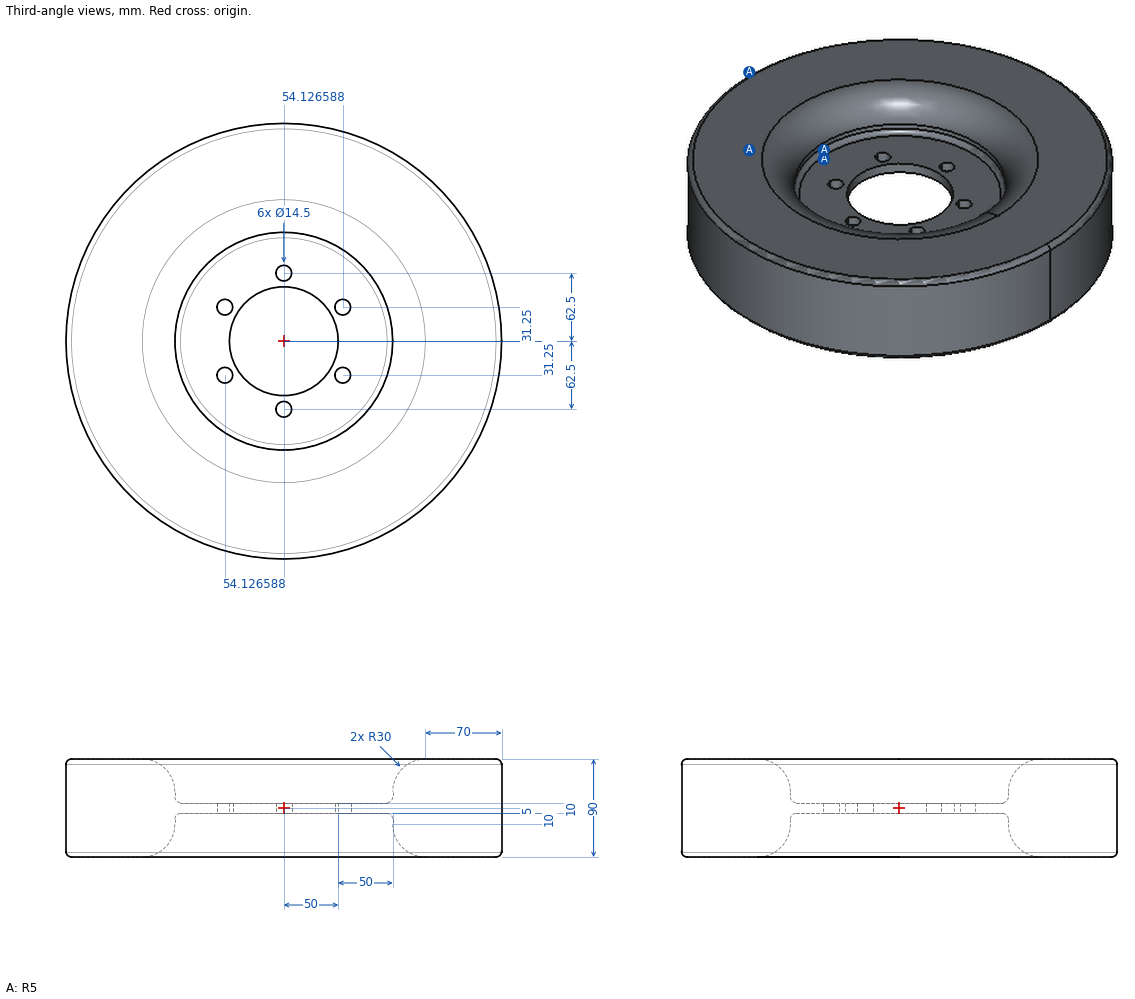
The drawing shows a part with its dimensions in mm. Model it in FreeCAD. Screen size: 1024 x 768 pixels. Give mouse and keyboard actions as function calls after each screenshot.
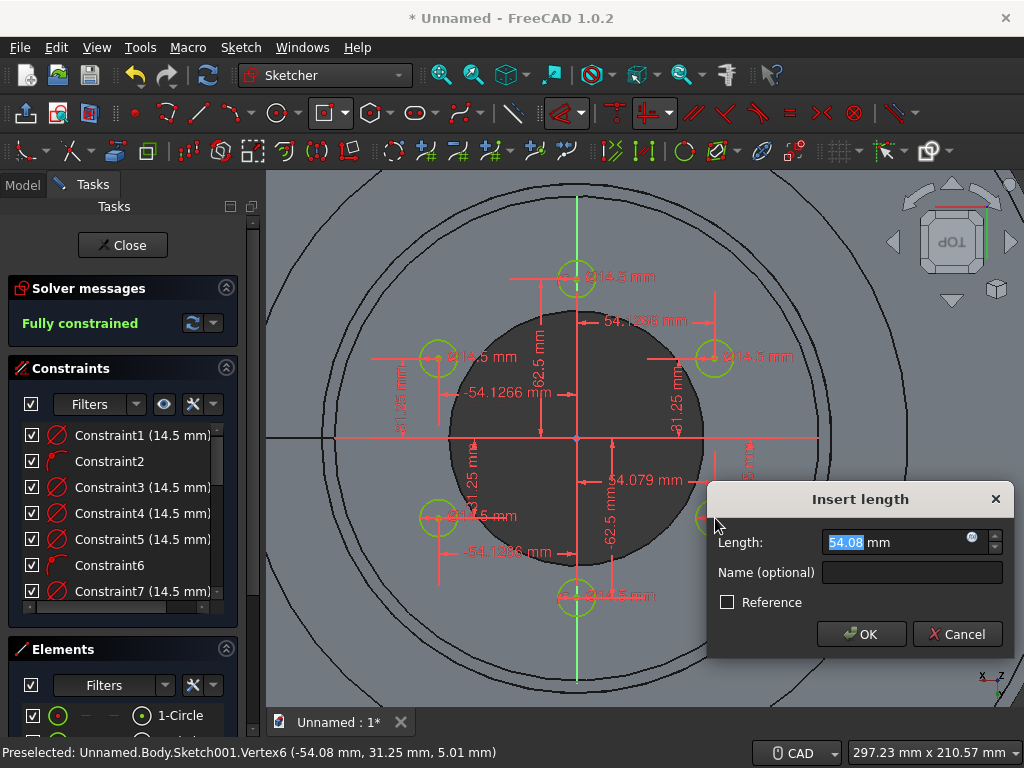
text(54.126588)
key(Return)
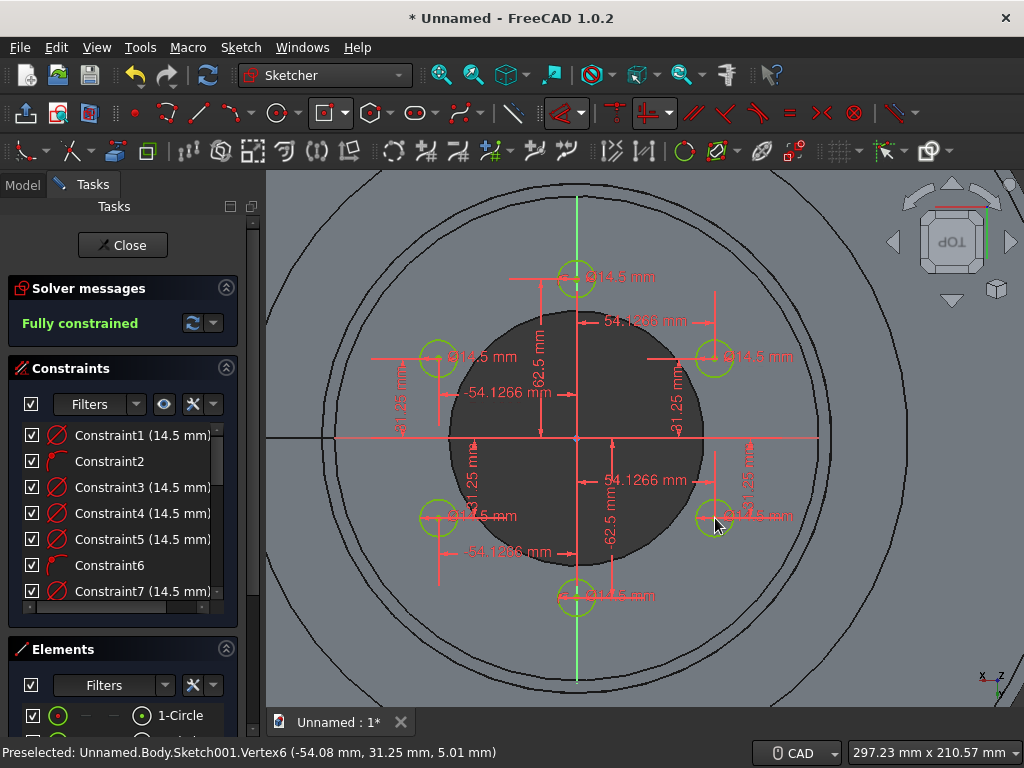
click(123, 245)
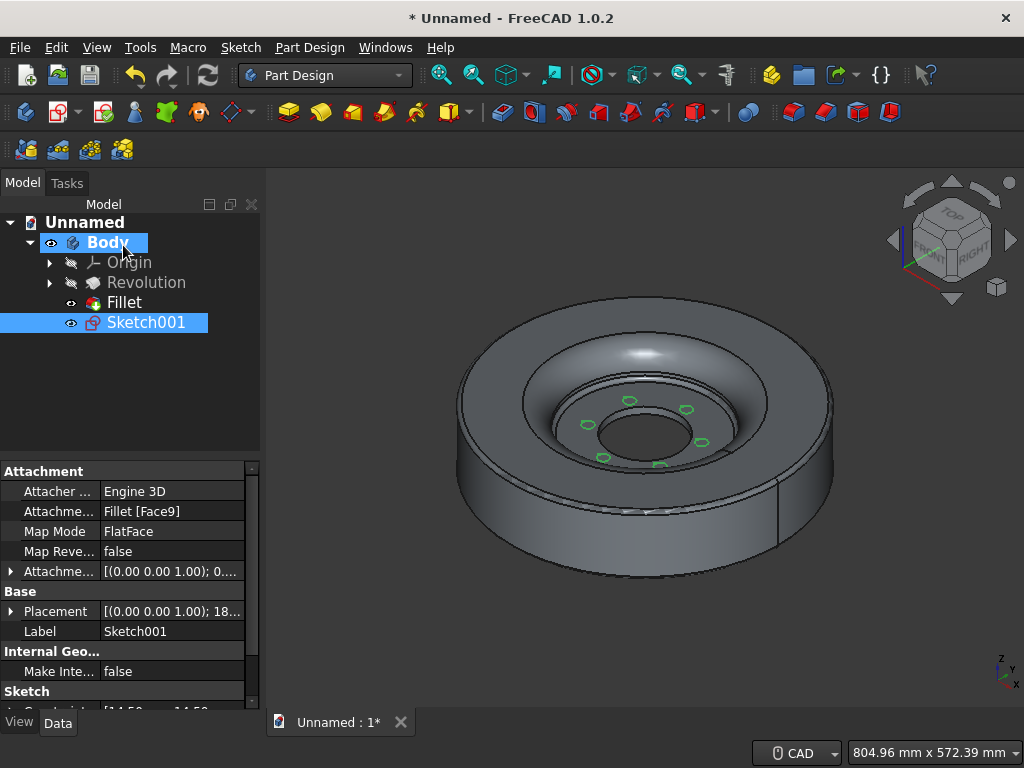
click(504, 112)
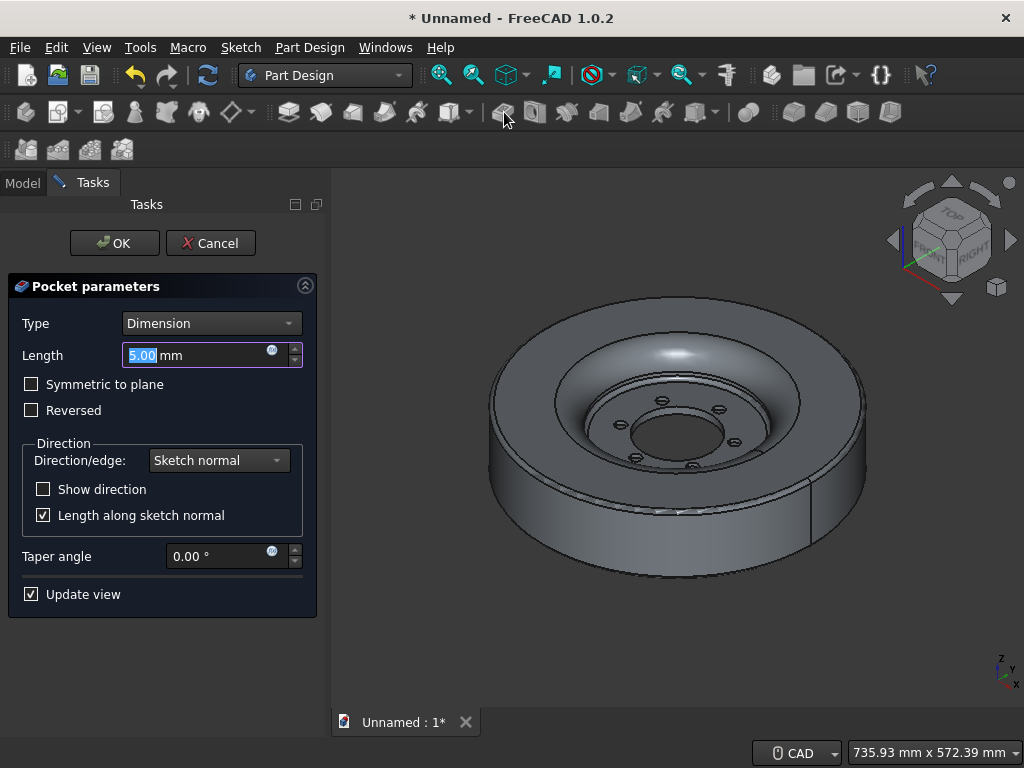
click(212, 324)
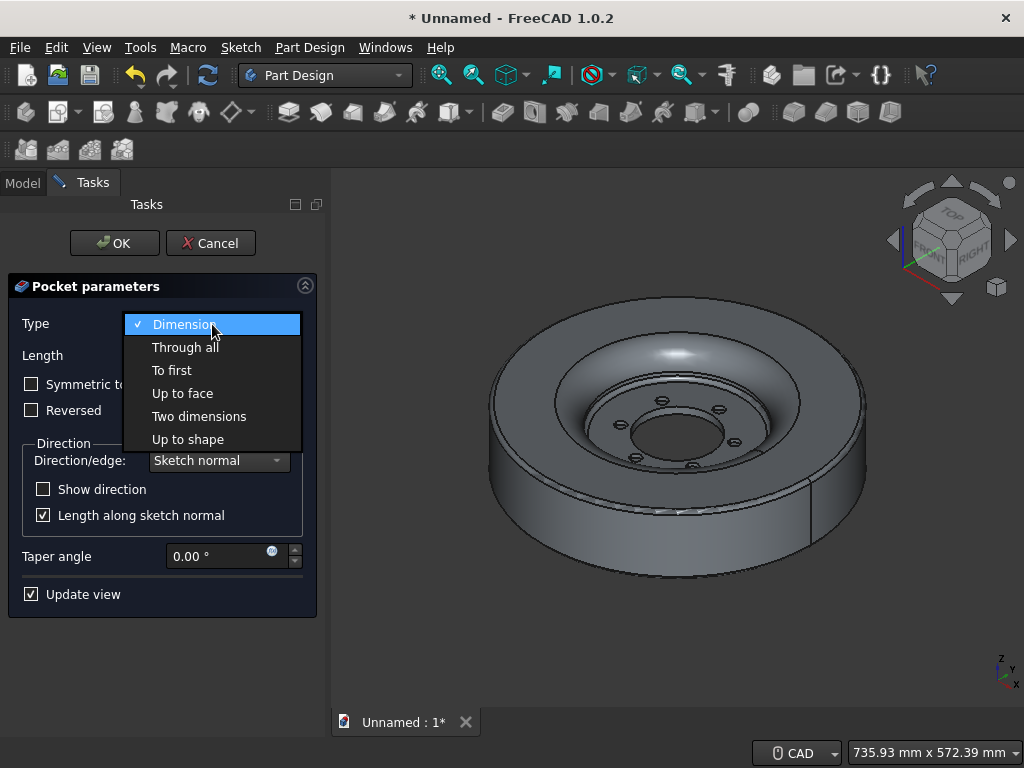
click(212, 348)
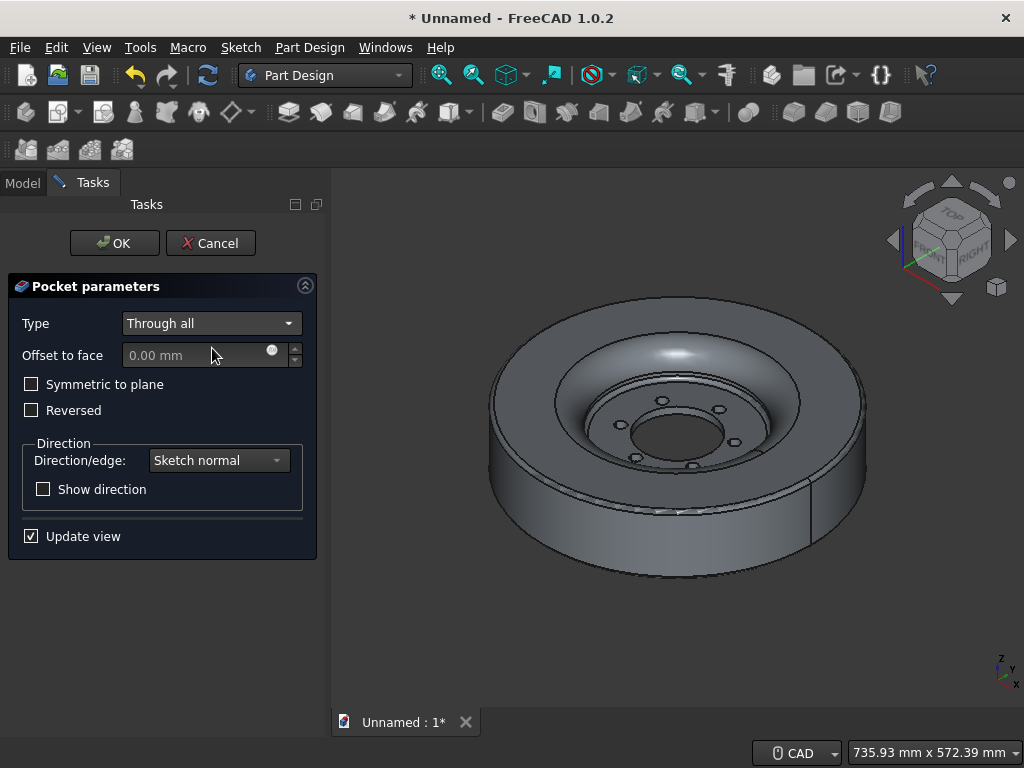
click(115, 243)